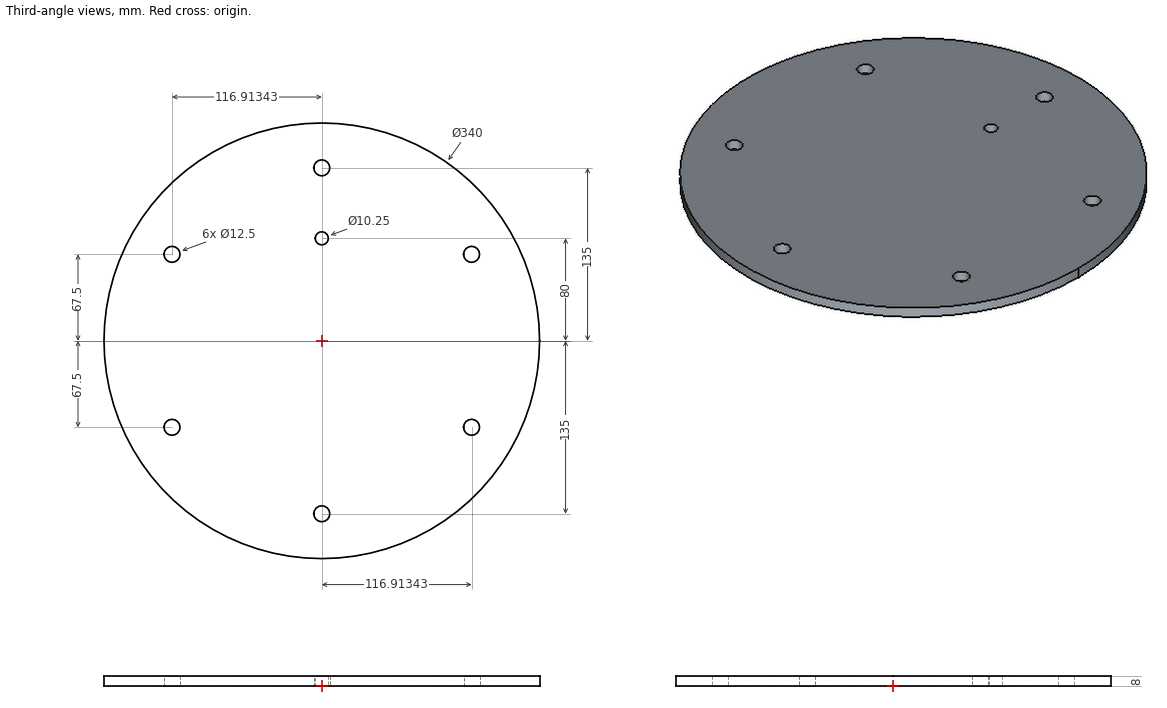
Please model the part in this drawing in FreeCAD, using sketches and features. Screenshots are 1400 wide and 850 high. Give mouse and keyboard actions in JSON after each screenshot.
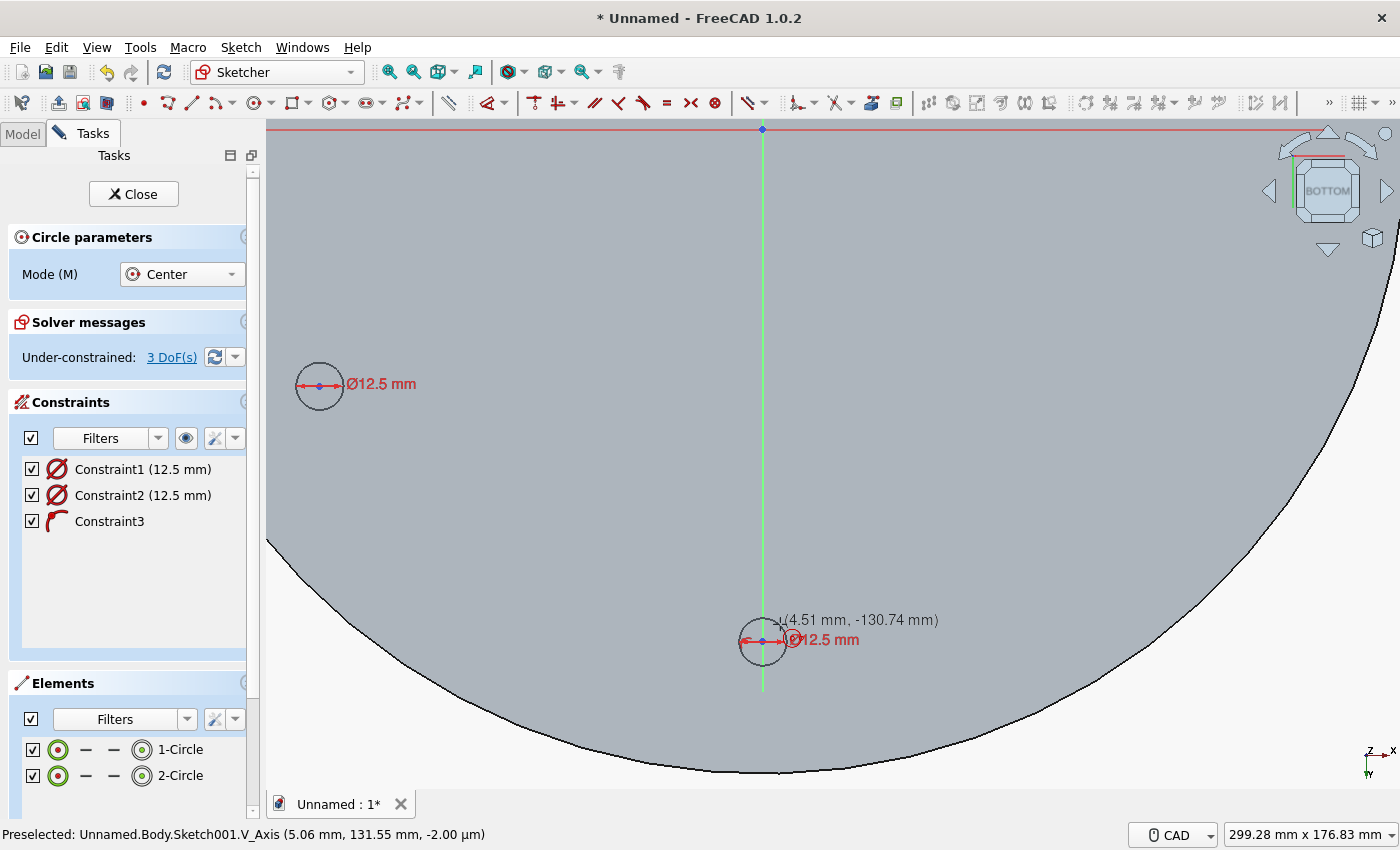
{"action": "scroll", "coordinate": [765, 643], "scroll_direction": "down", "scroll_amount": 5}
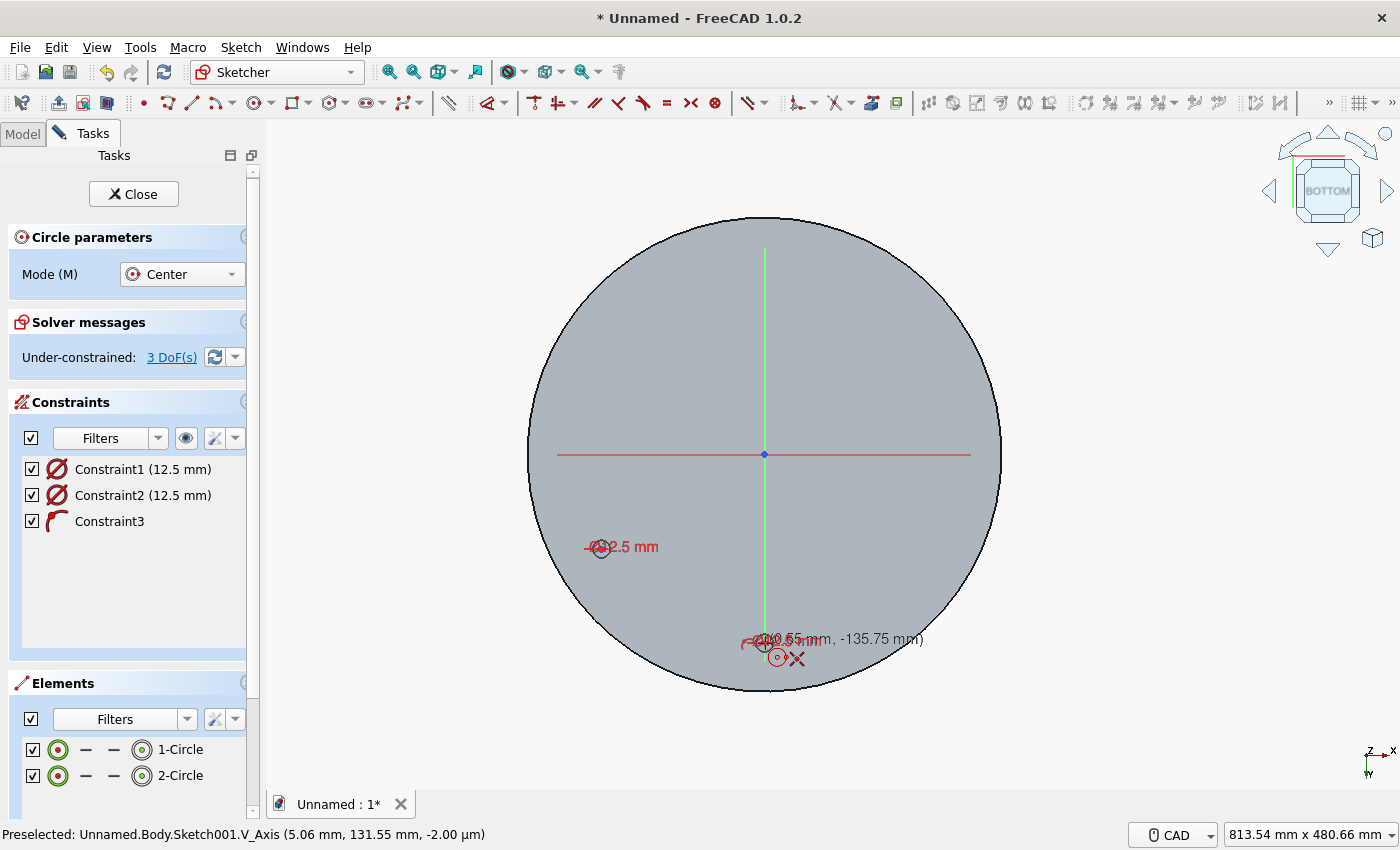
{"action": "scroll", "coordinate": [602, 361], "scroll_direction": "up", "scroll_amount": 5}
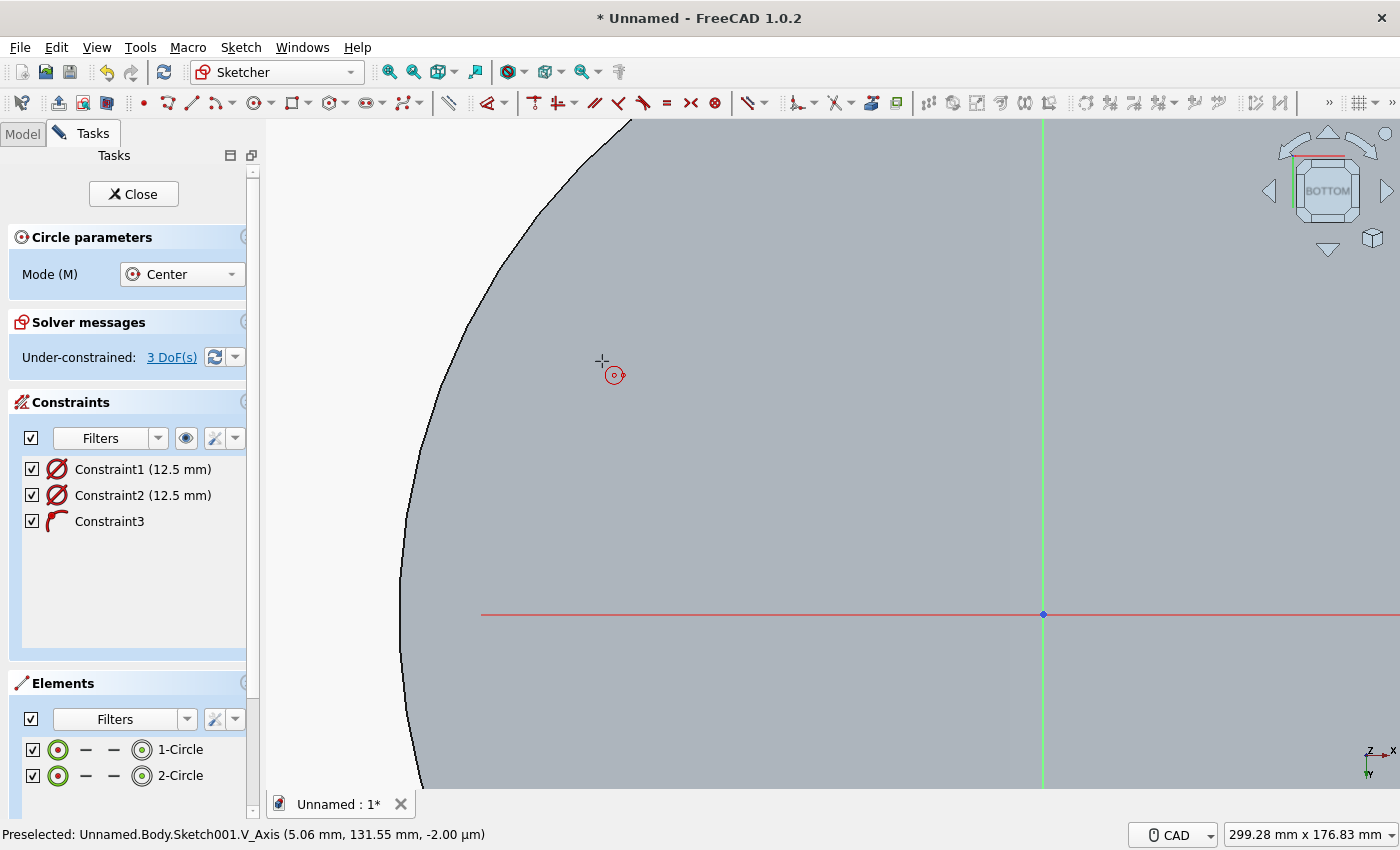
{"action": "left_click", "coordinate": [600, 359]}
{"action": "mouse_move", "coordinate": [617, 342]}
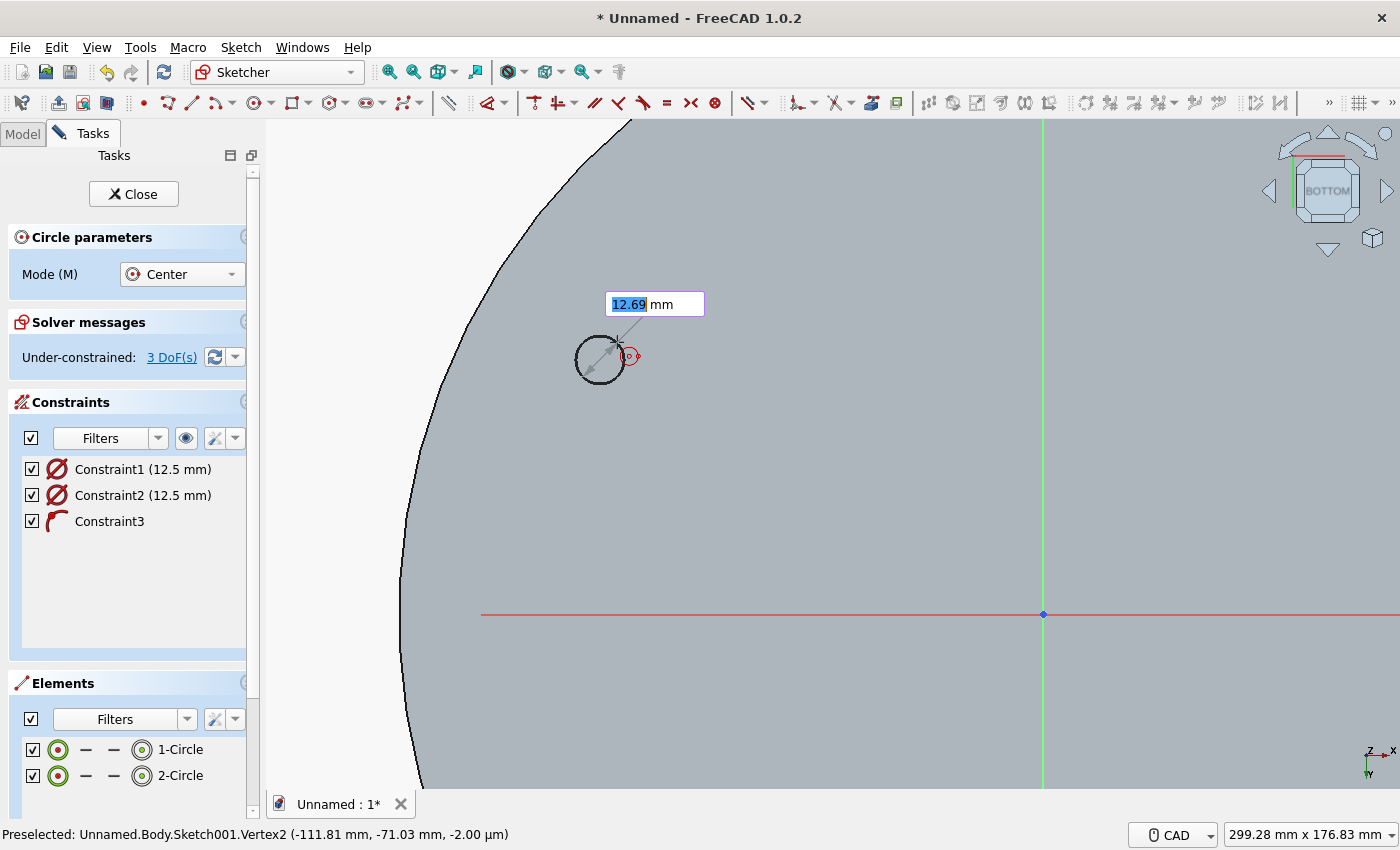
{"action": "type", "text": "12.5"}
{"action": "key", "text": "Return"}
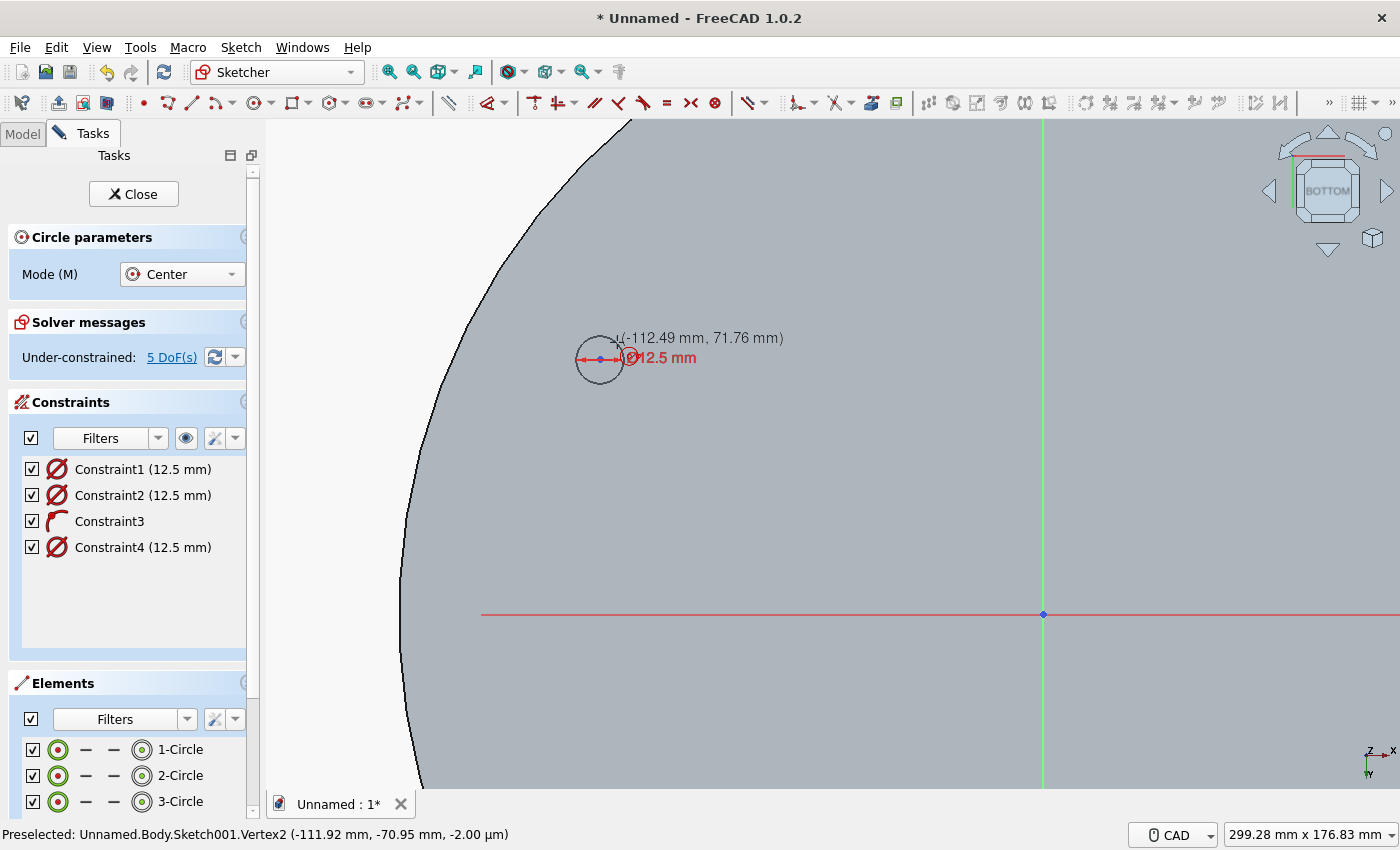
{"action": "scroll", "coordinate": [602, 360], "scroll_direction": "down", "scroll_amount": 5}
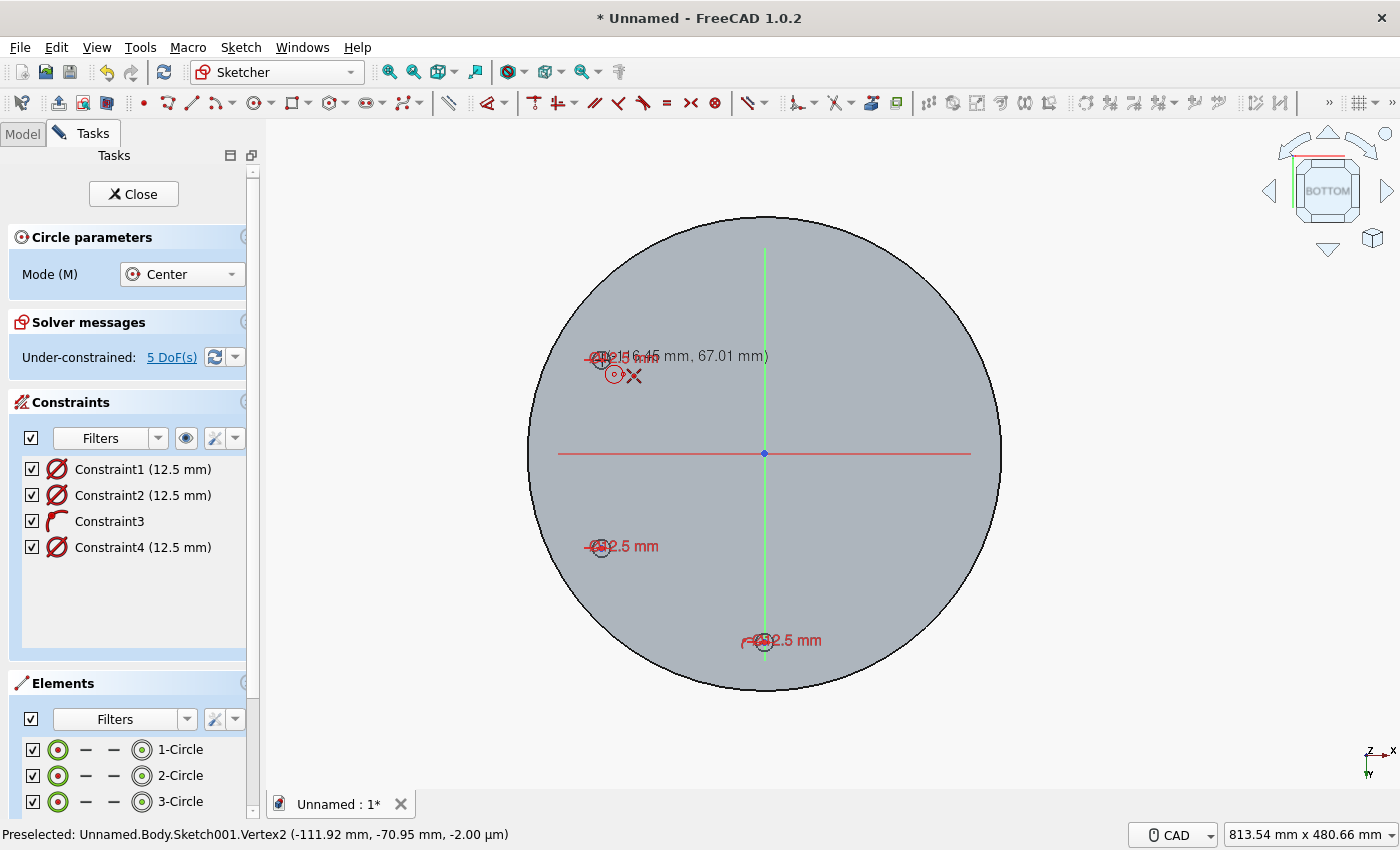
{"action": "scroll", "coordinate": [765, 266], "scroll_direction": "up", "scroll_amount": 5}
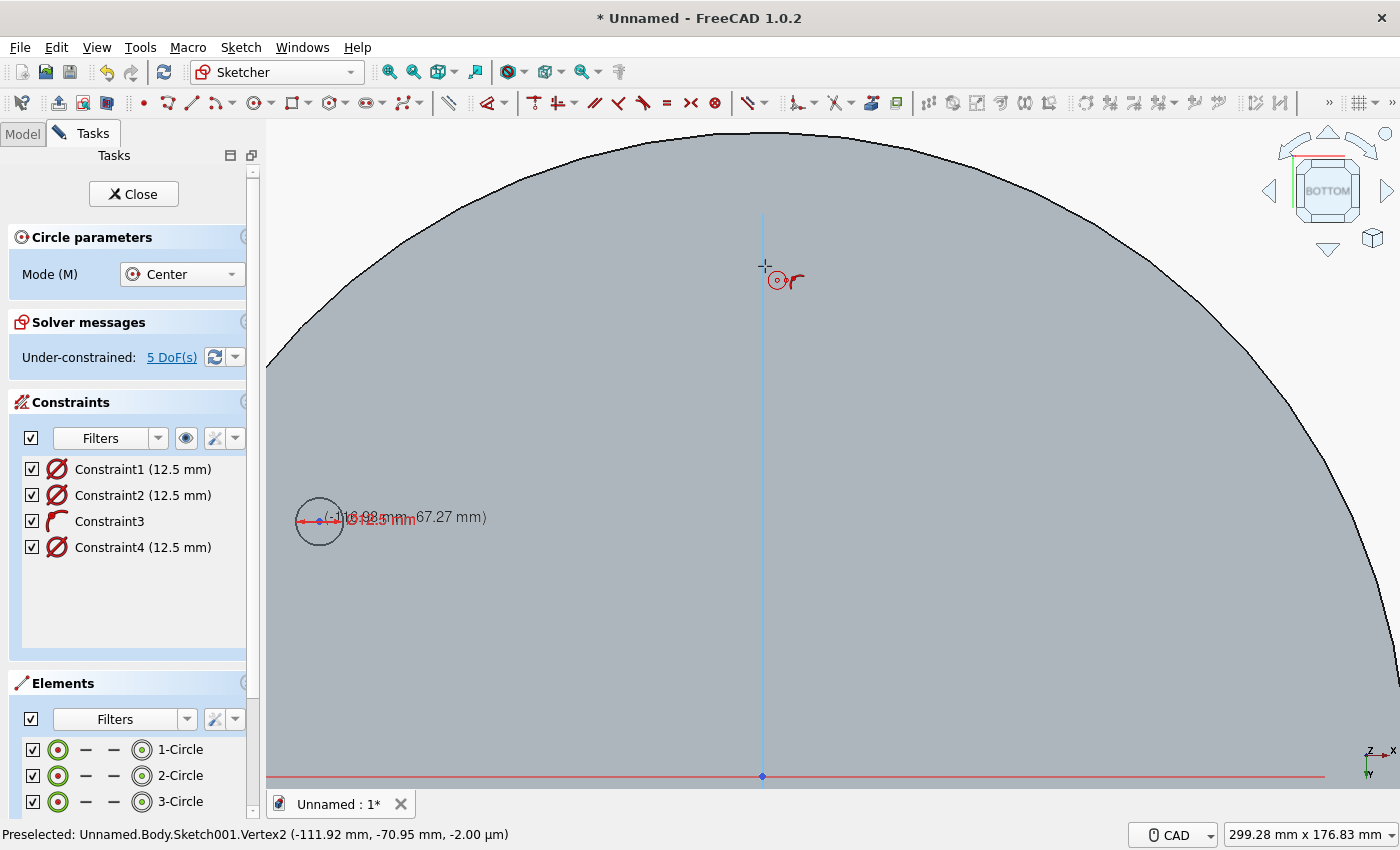
{"action": "left_click", "coordinate": [763, 265]}
{"action": "mouse_move", "coordinate": [780, 248]}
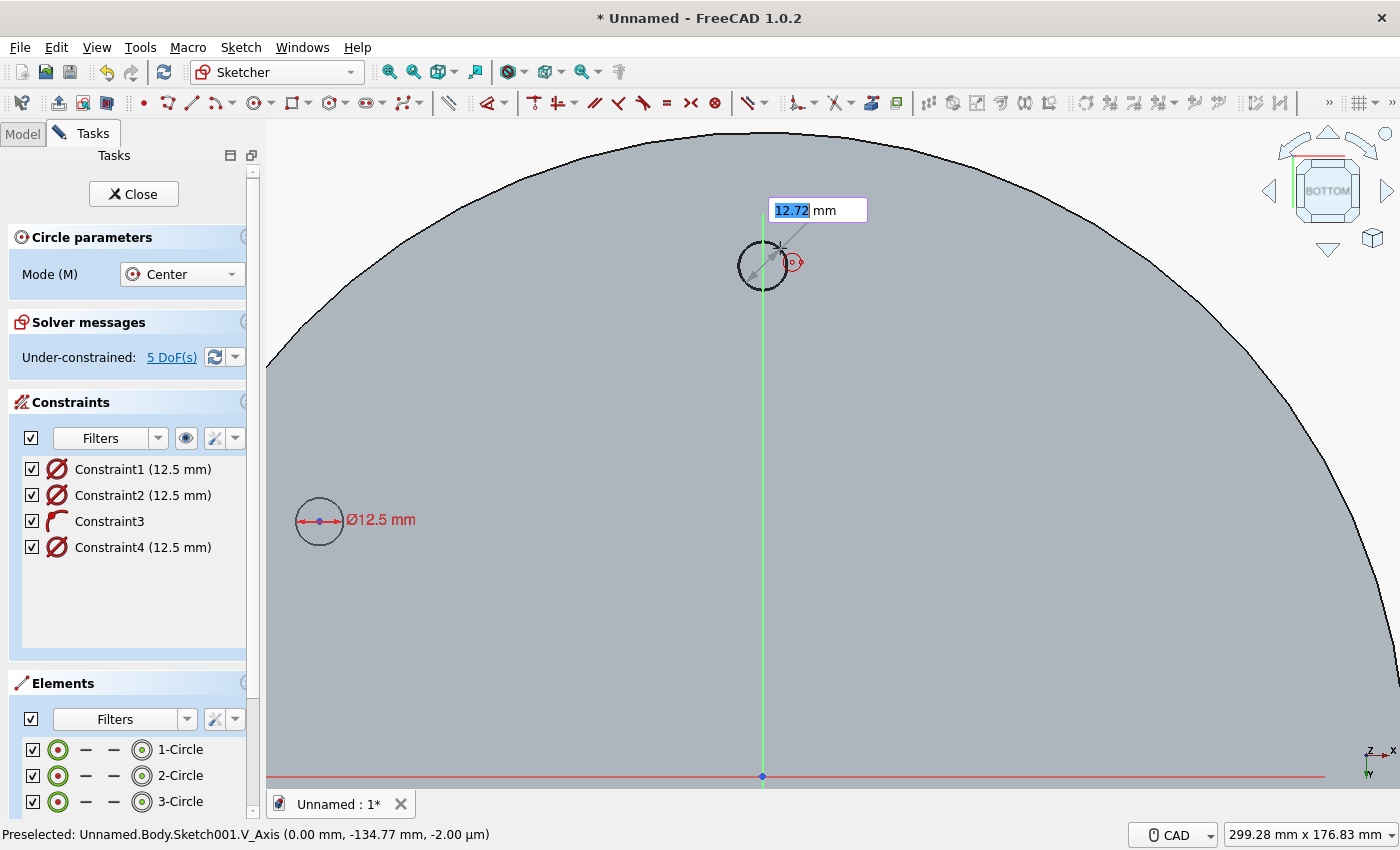
{"action": "type", "text": "12.5"}
{"action": "key", "text": "Return"}